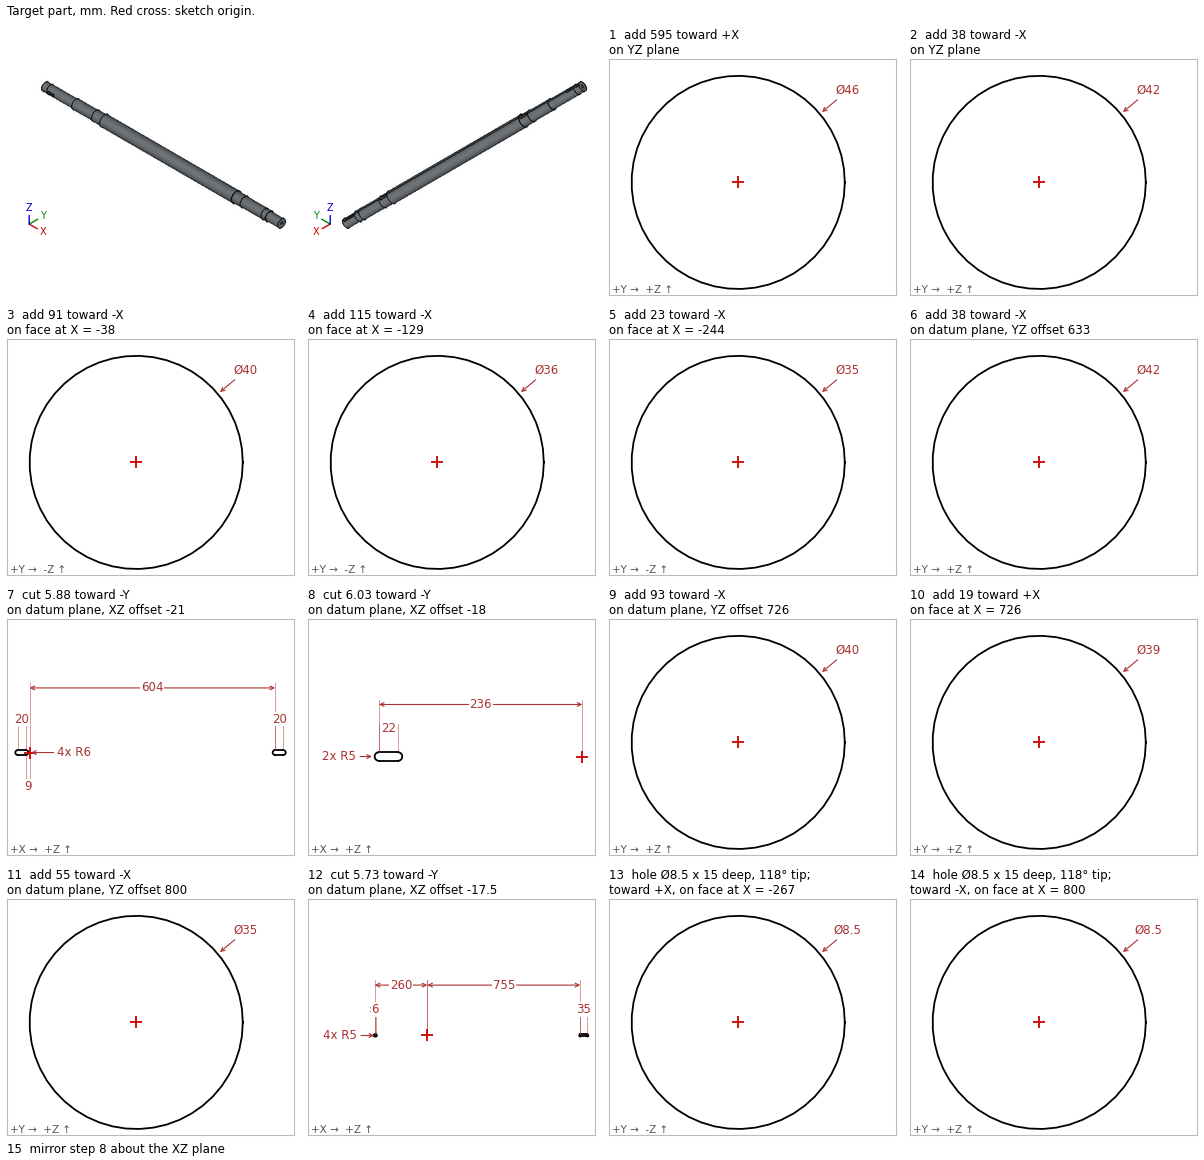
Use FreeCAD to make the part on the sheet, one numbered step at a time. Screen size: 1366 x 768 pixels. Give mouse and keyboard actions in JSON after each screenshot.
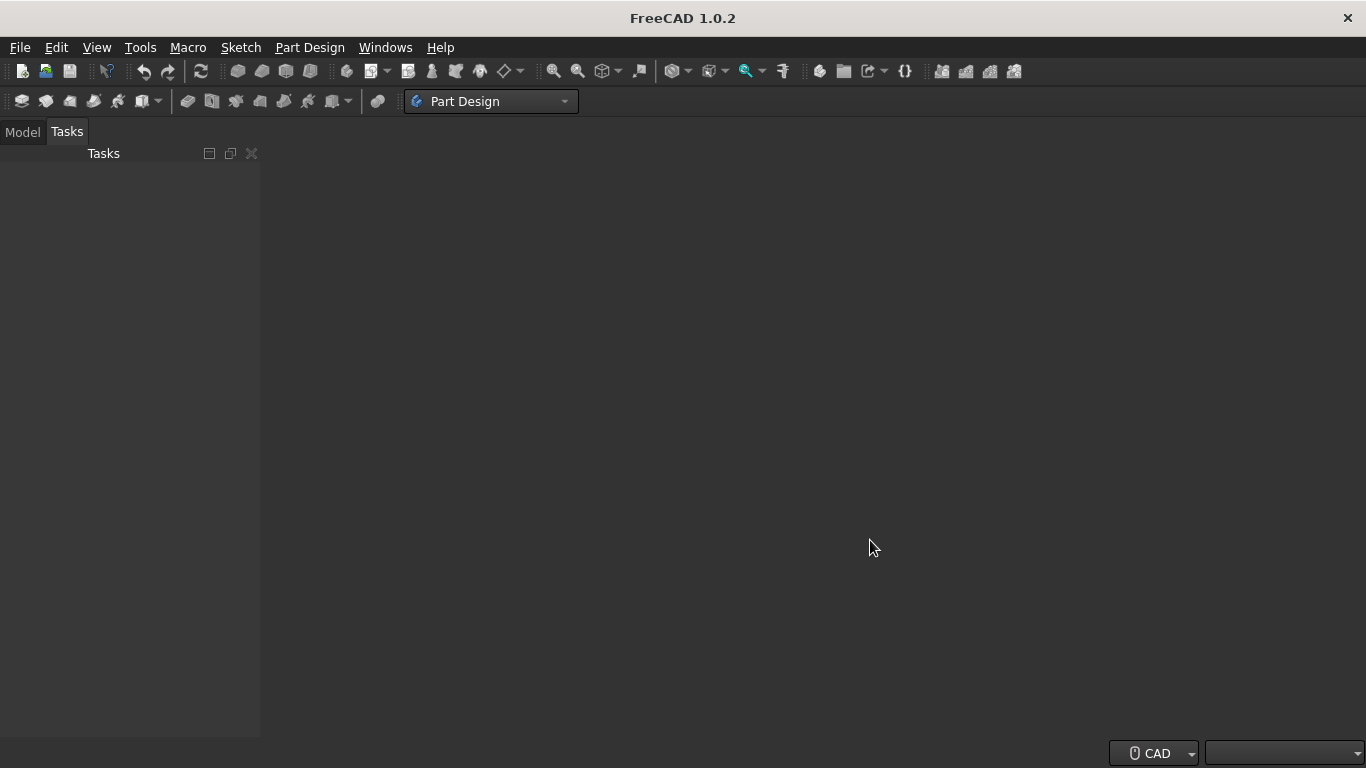
{"action": "key", "text": "ctrl+n"}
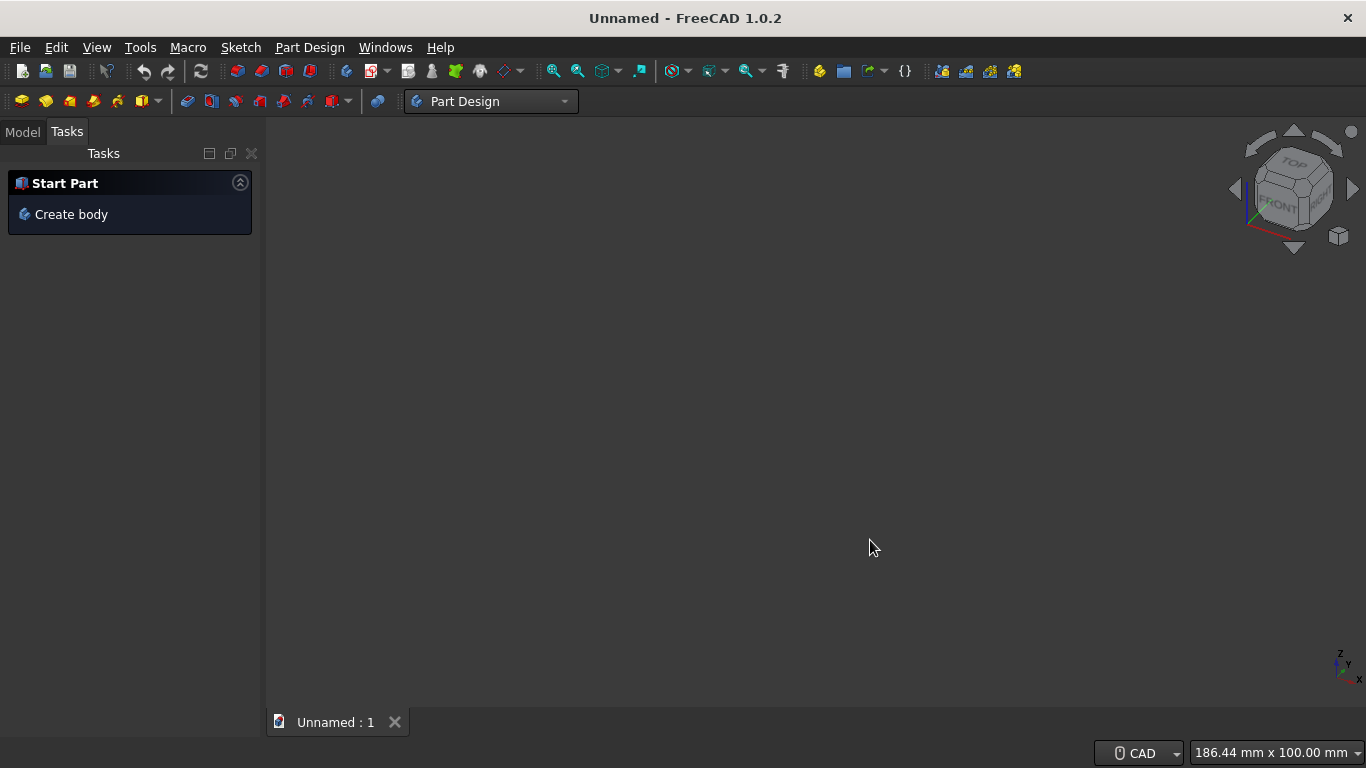
{"action": "left_click", "coordinate": [372, 72]}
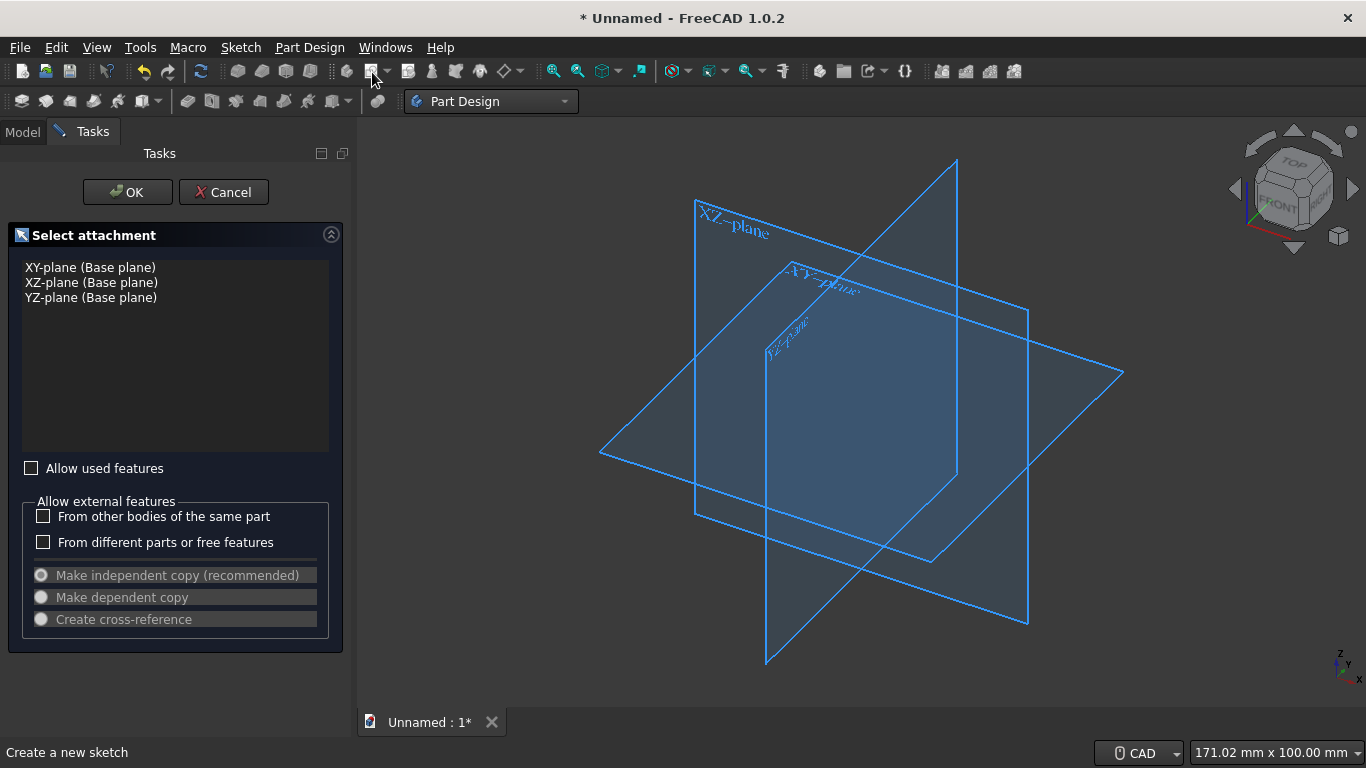
{"action": "left_click", "coordinate": [82, 298]}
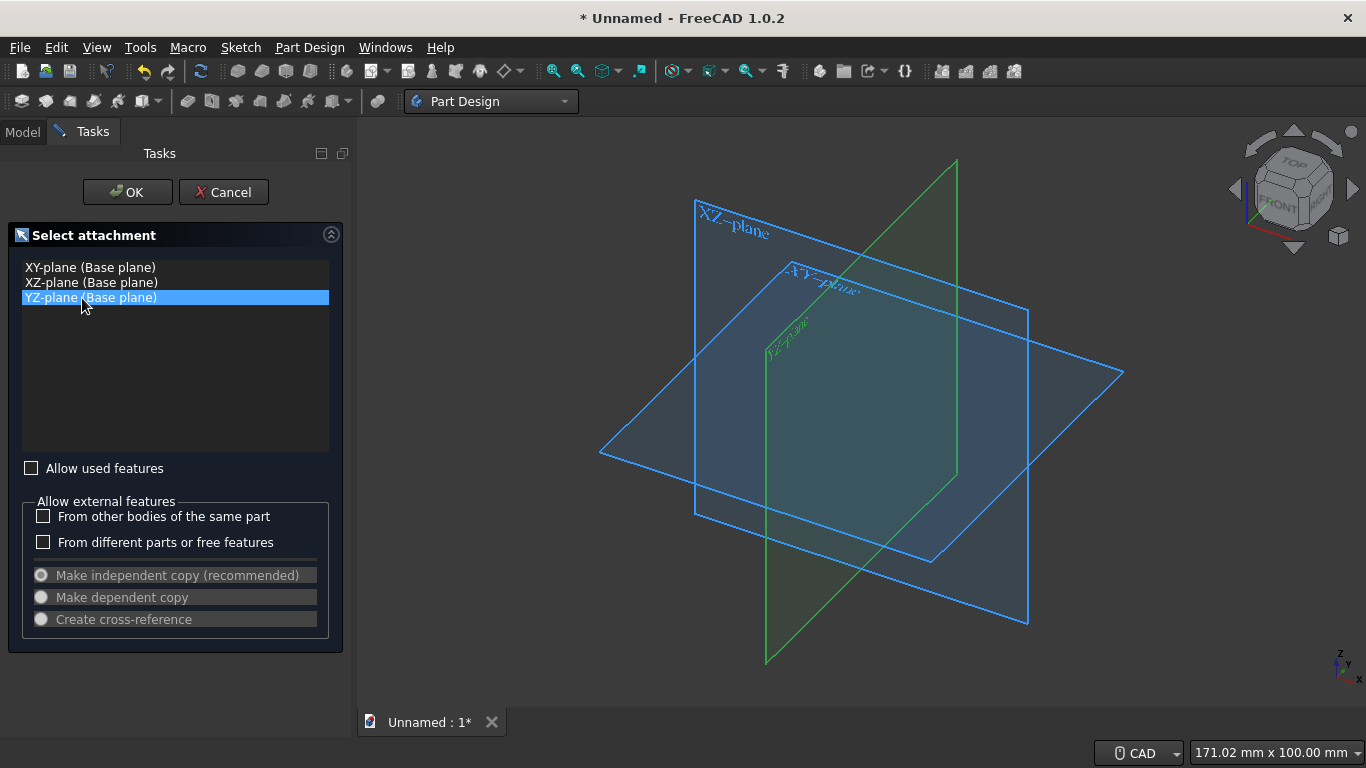
{"action": "left_click", "coordinate": [128, 192]}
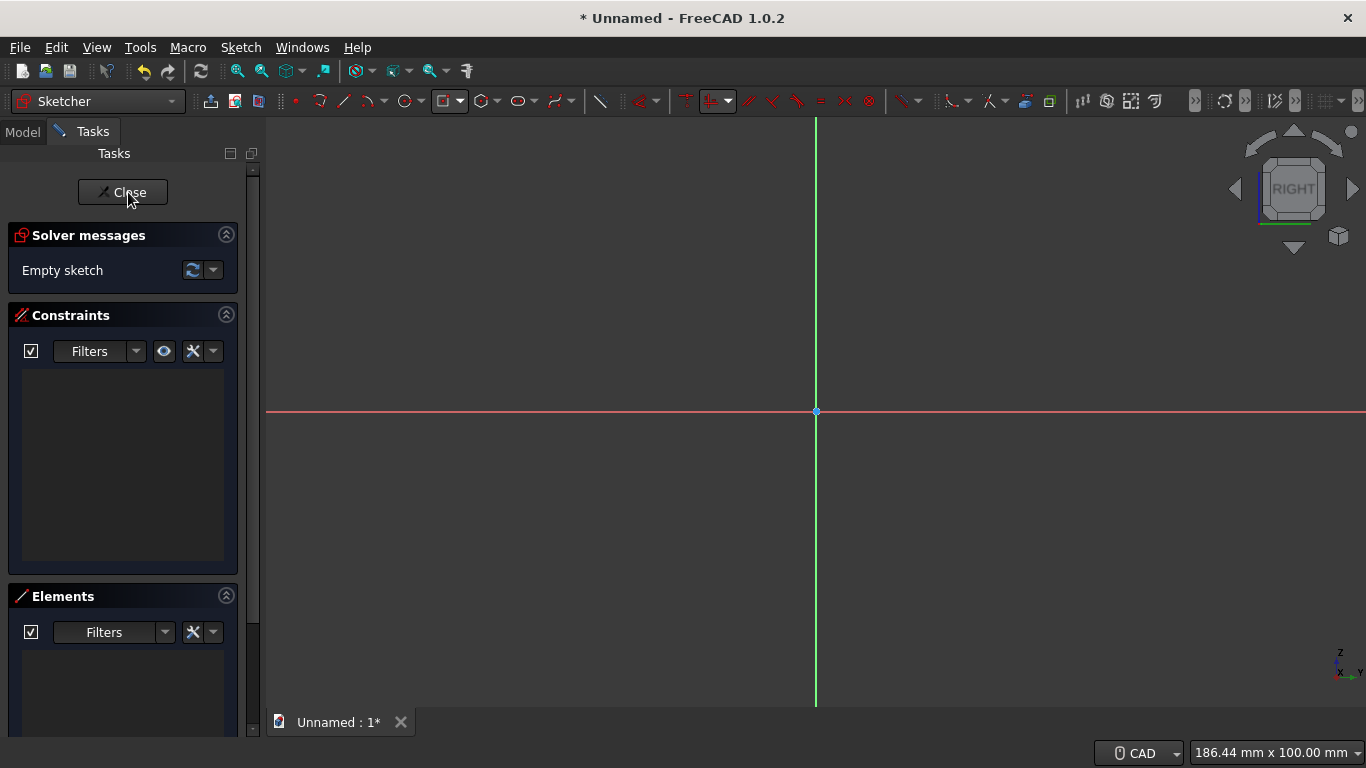
{"action": "scroll", "coordinate": [955, 412], "scroll_direction": "up", "scroll_amount": 2}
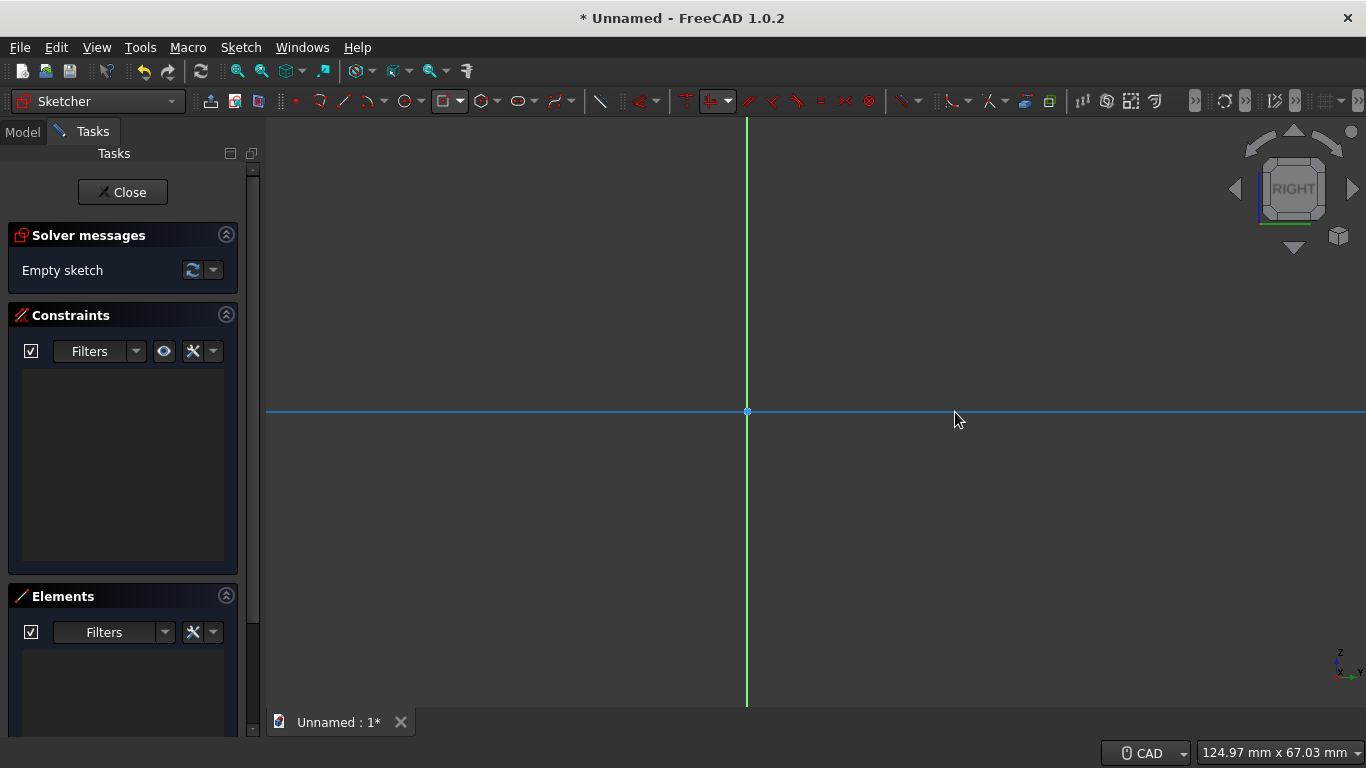
{"action": "key", "text": "g c"}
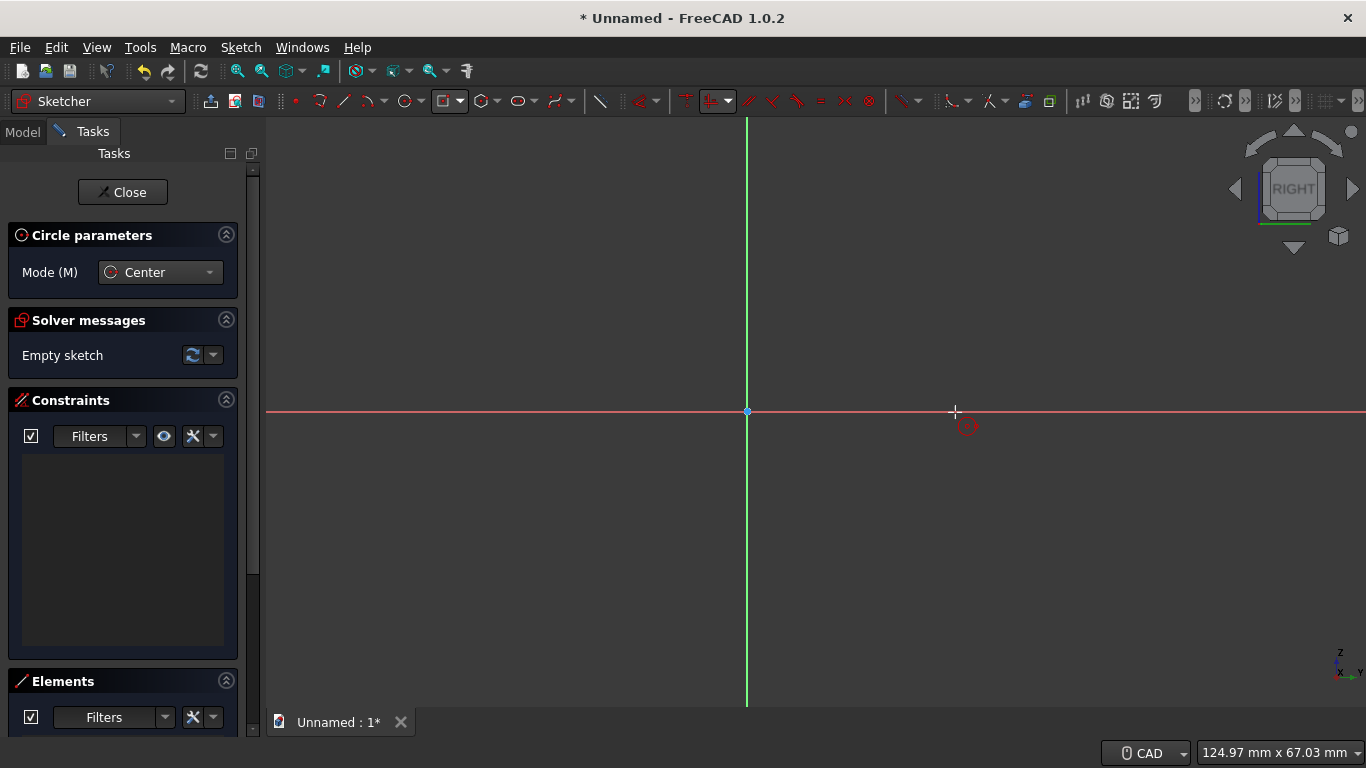
{"action": "left_click", "coordinate": [747, 412]}
{"action": "mouse_move", "coordinate": [890, 269]}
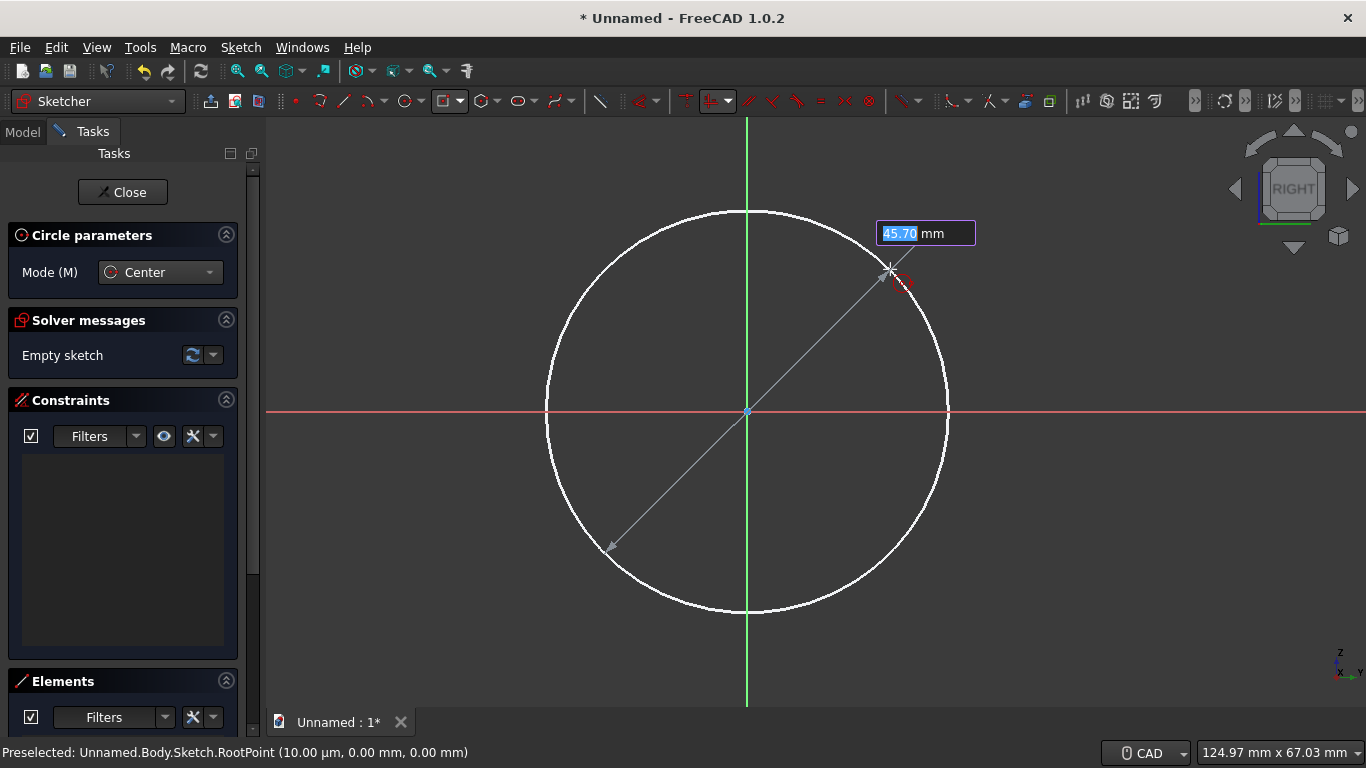
{"action": "type", "text": "46"}
{"action": "key", "text": "Return"}
{"action": "key", "text": "Escape"}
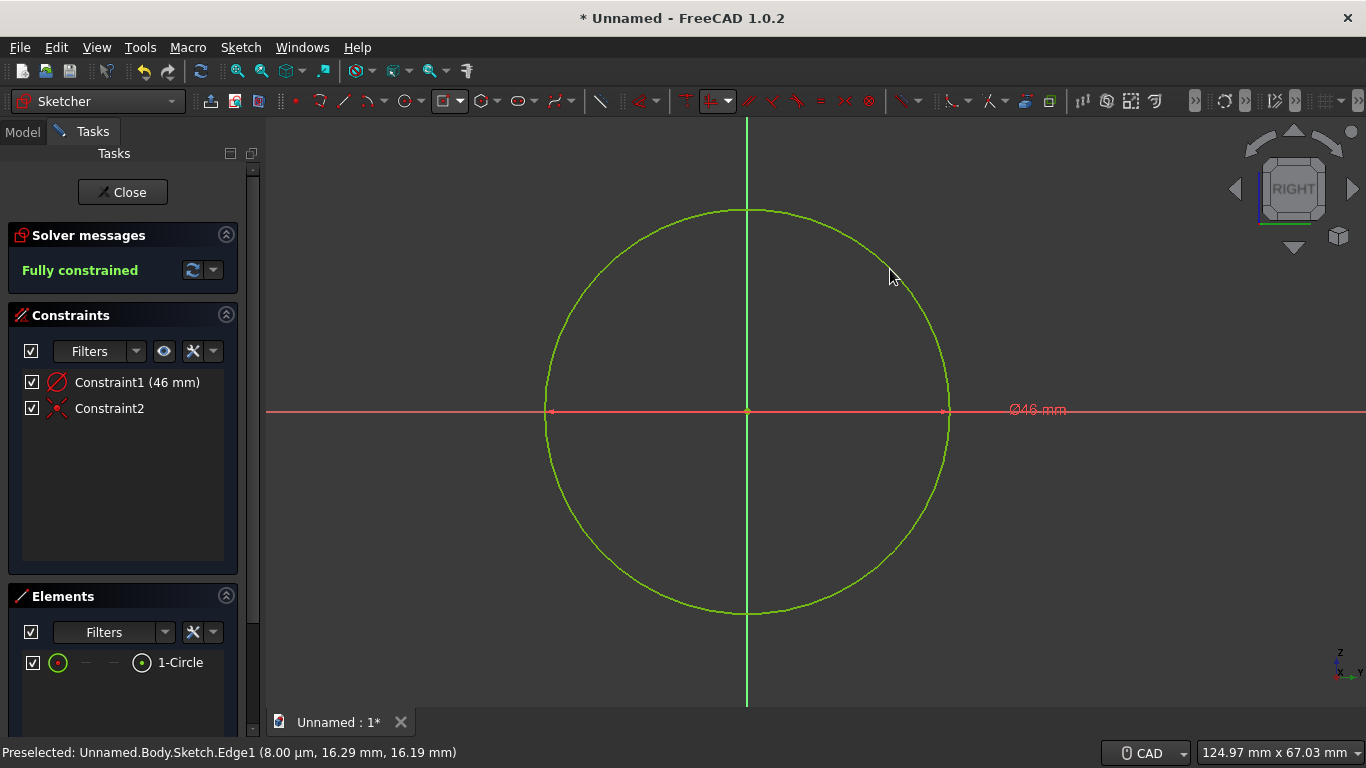
{"action": "left_click", "coordinate": [123, 192]}